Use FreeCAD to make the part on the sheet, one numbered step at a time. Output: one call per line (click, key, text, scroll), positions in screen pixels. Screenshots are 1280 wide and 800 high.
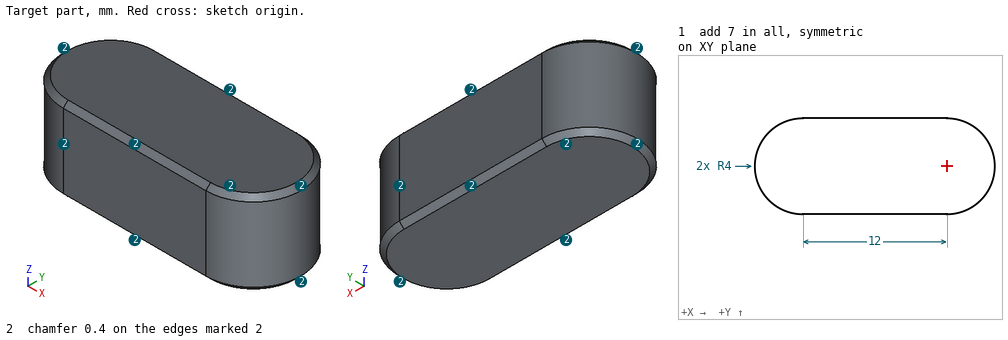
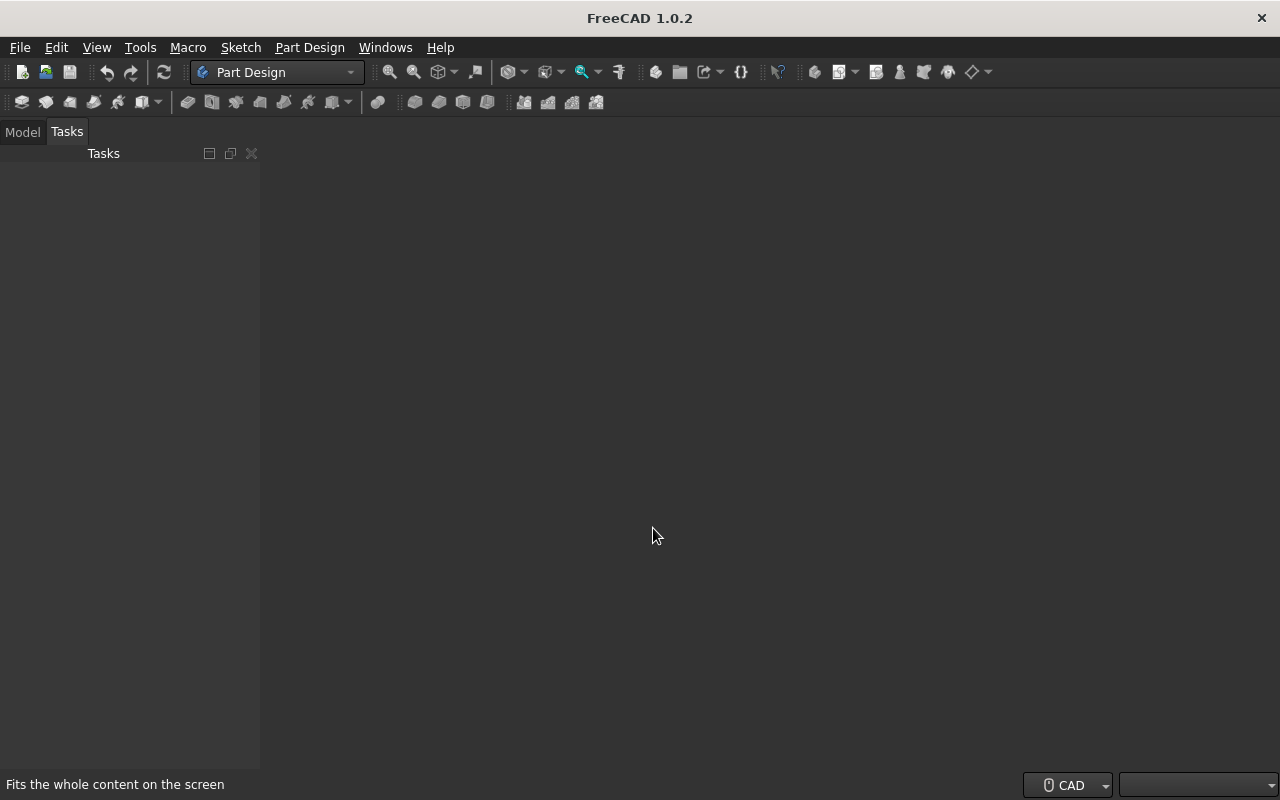
click(22, 72)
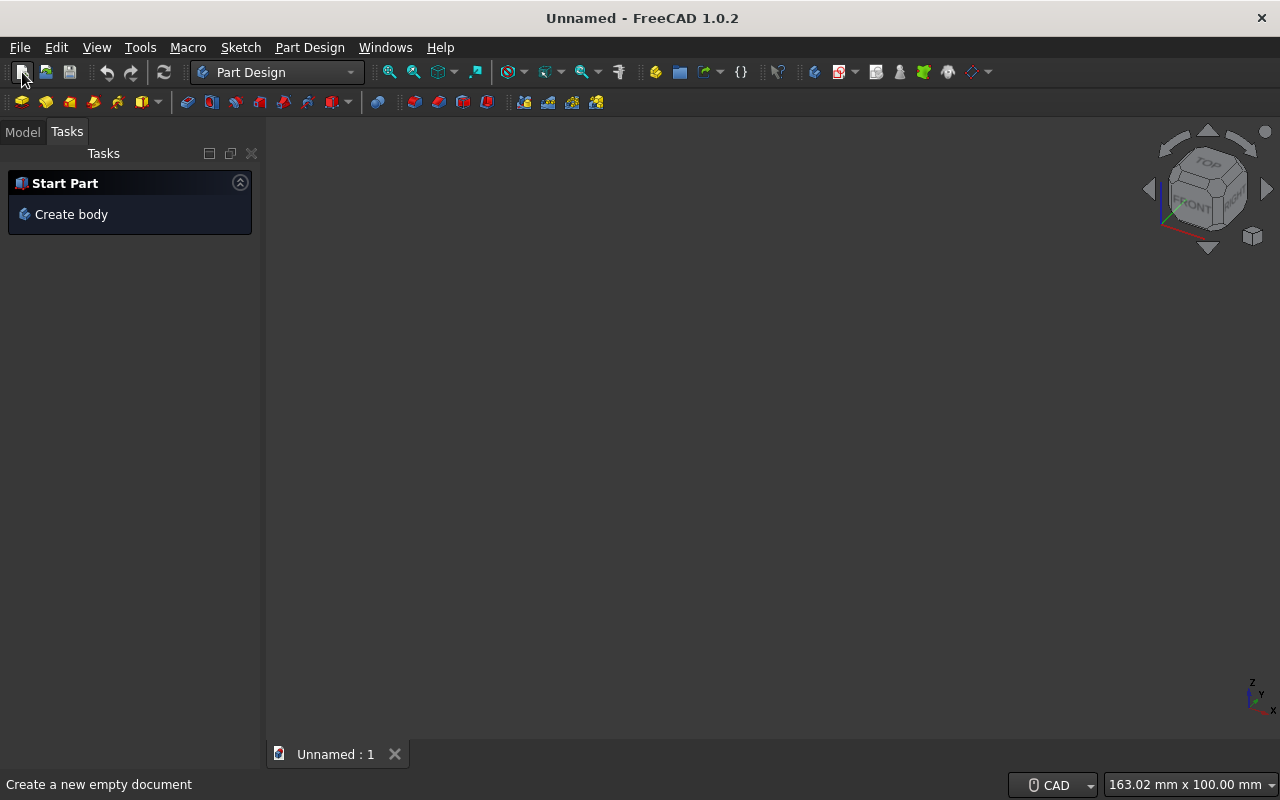
click(840, 72)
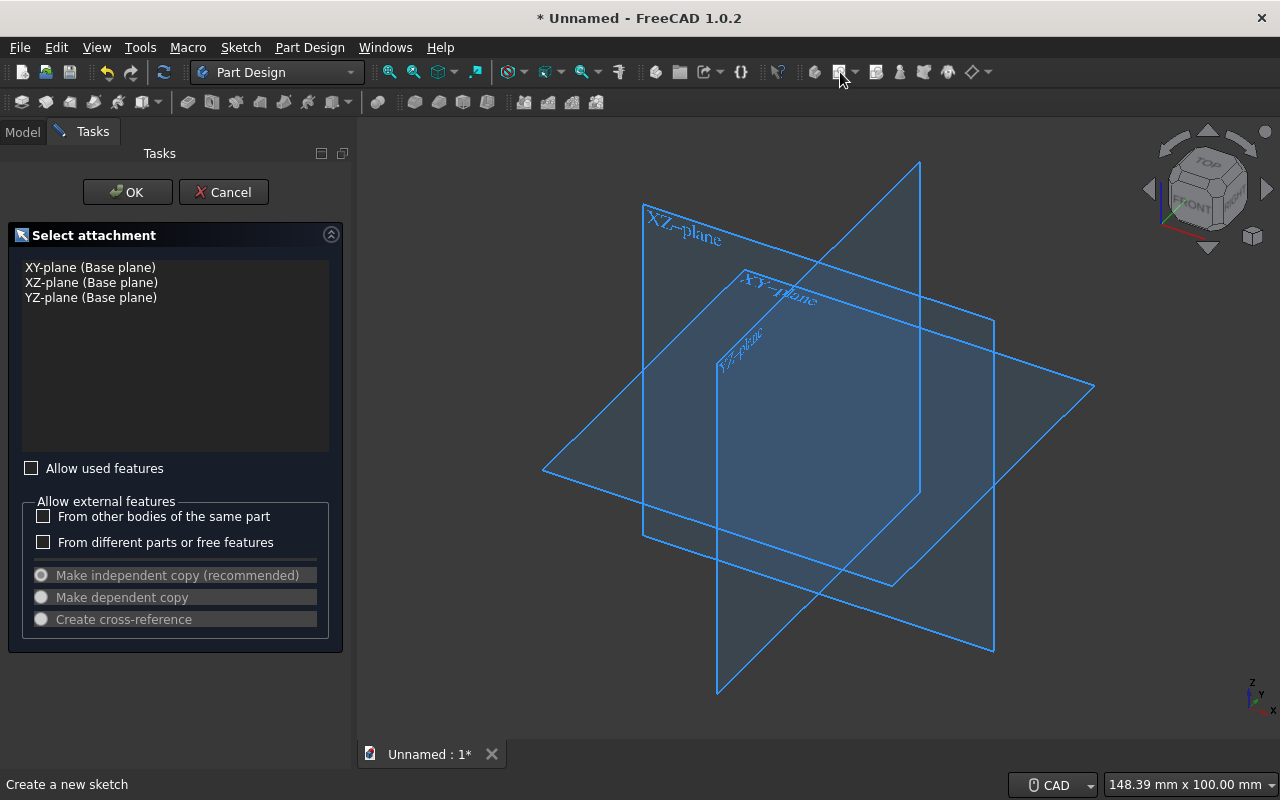
click(82, 268)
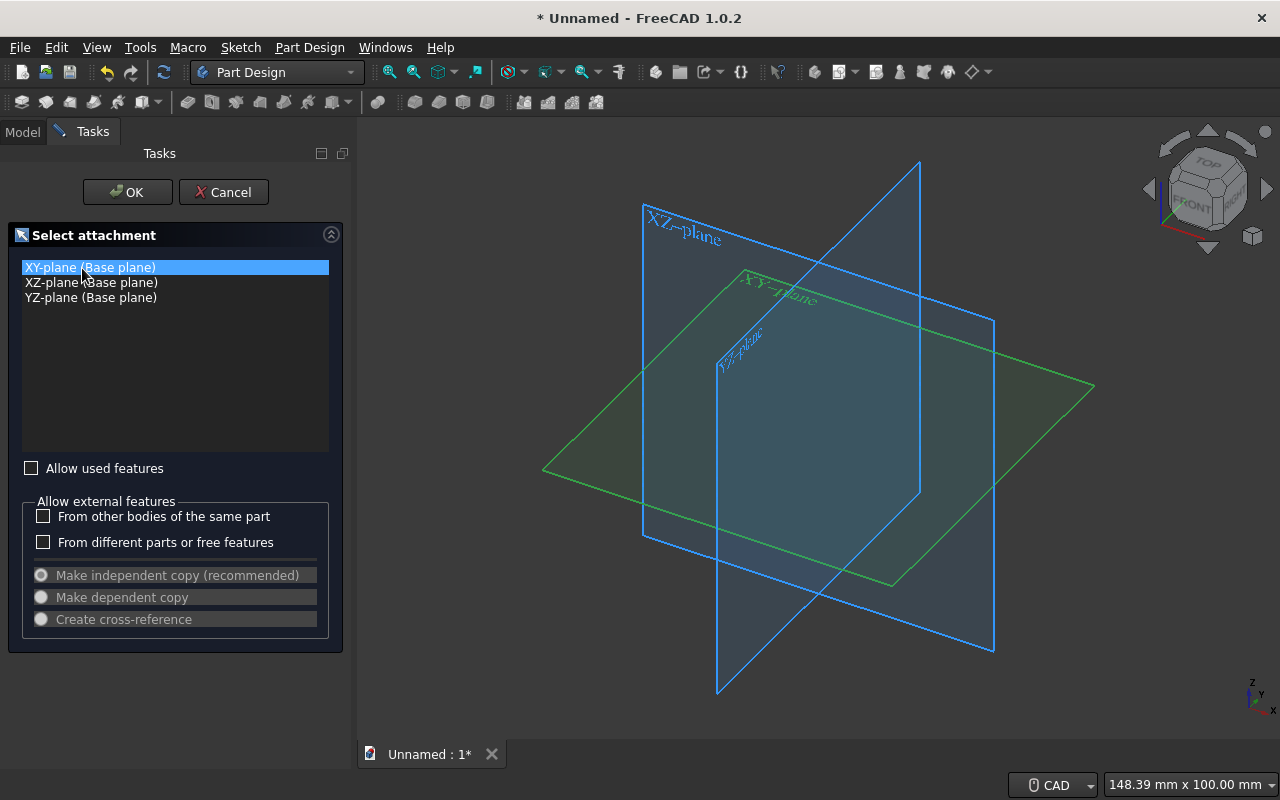
click(128, 192)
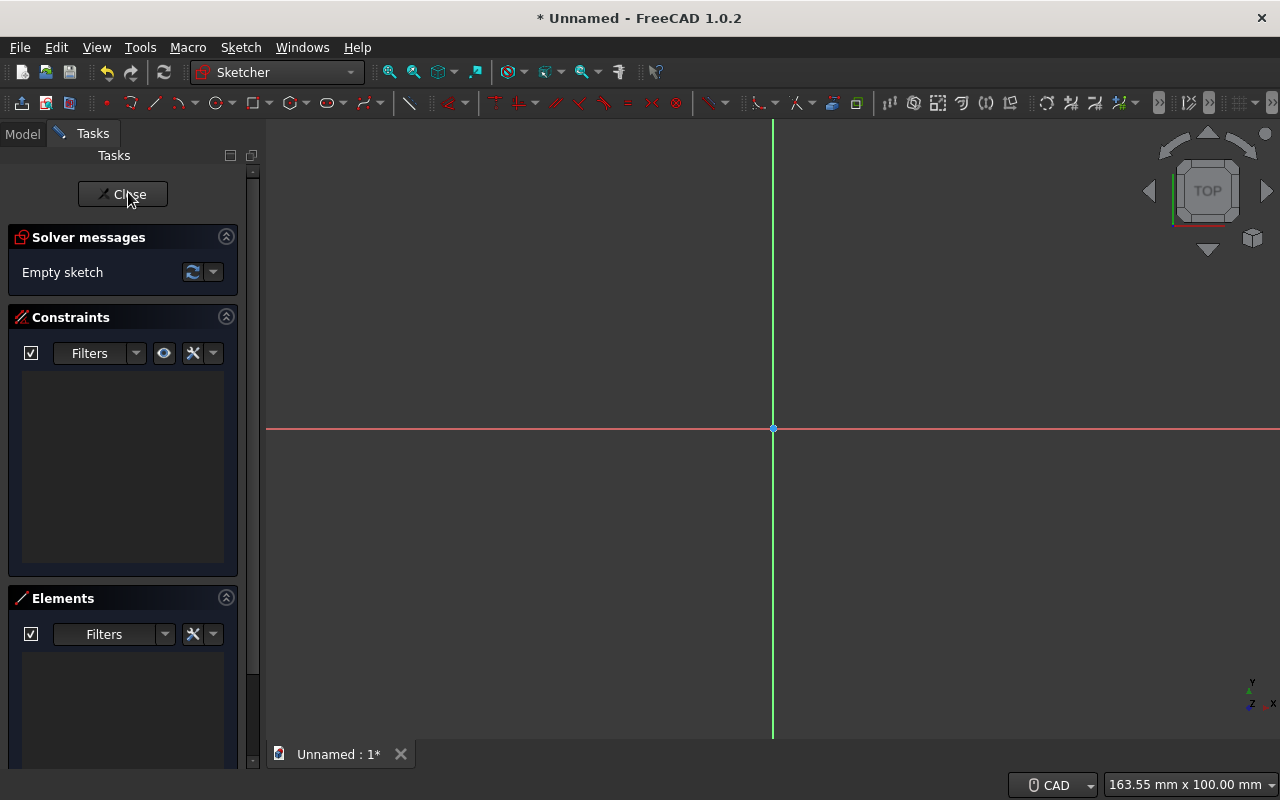
scroll(744, 429, up, 8)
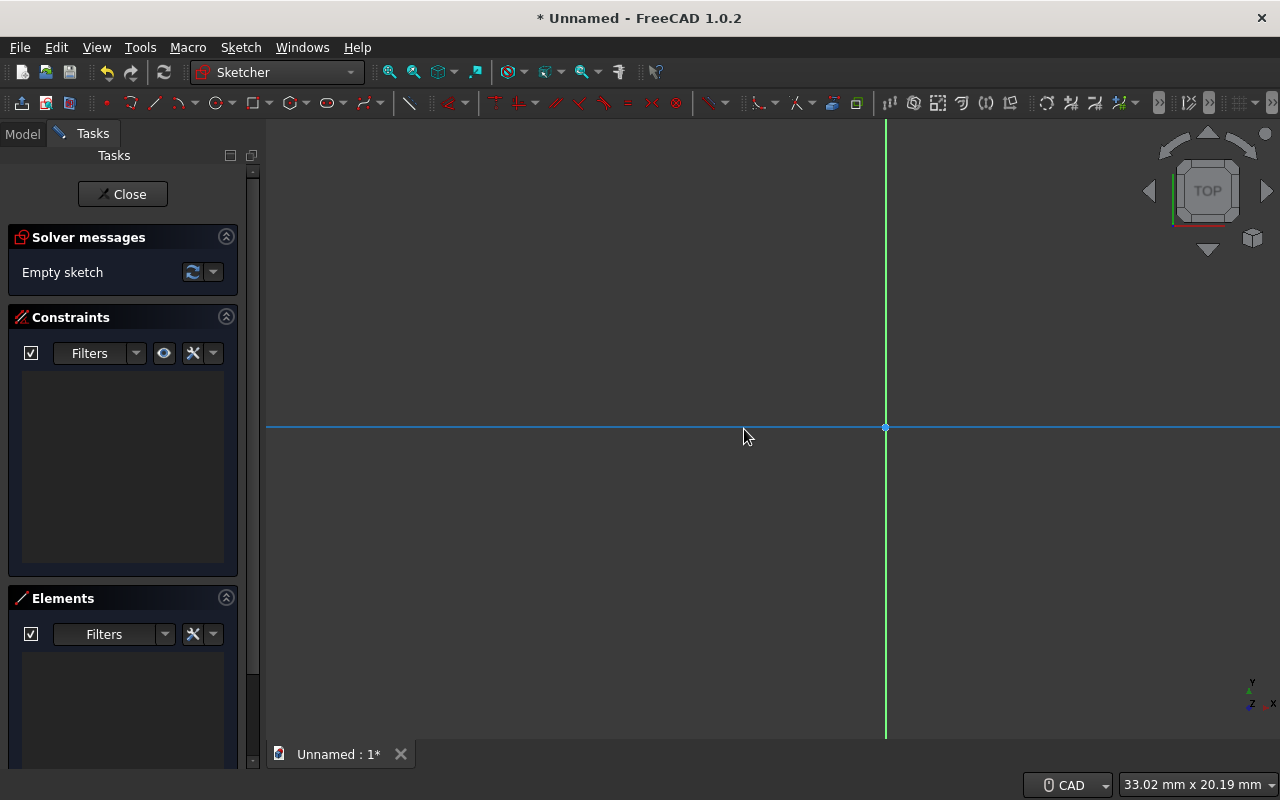
click(328, 104)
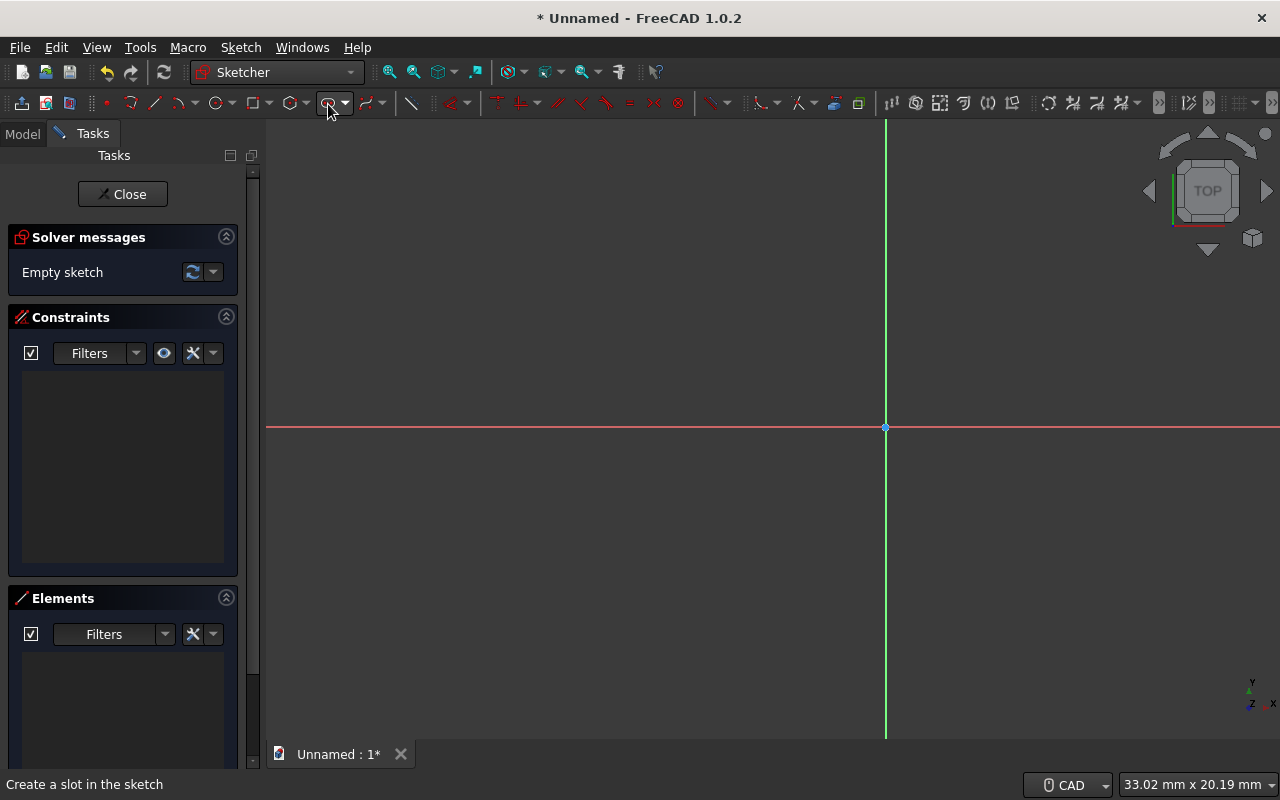
click(886, 427)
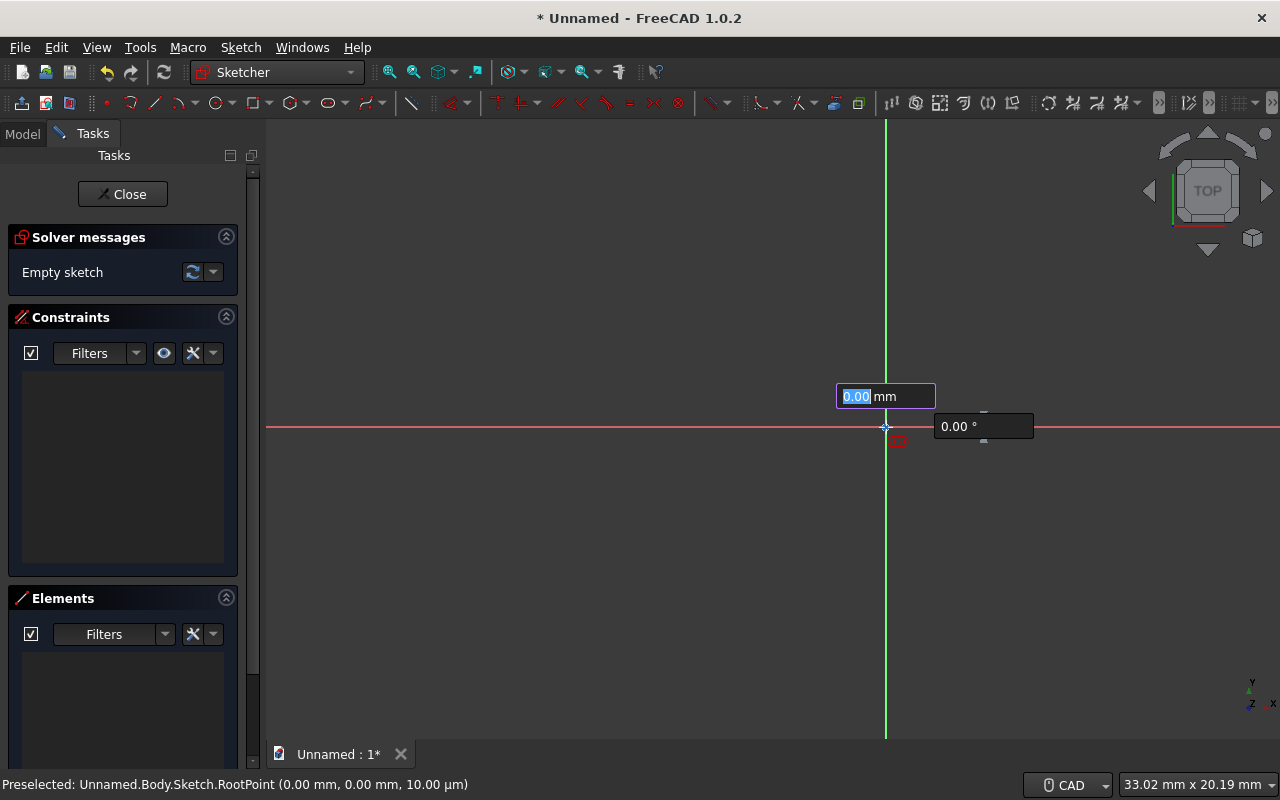
click(517, 418)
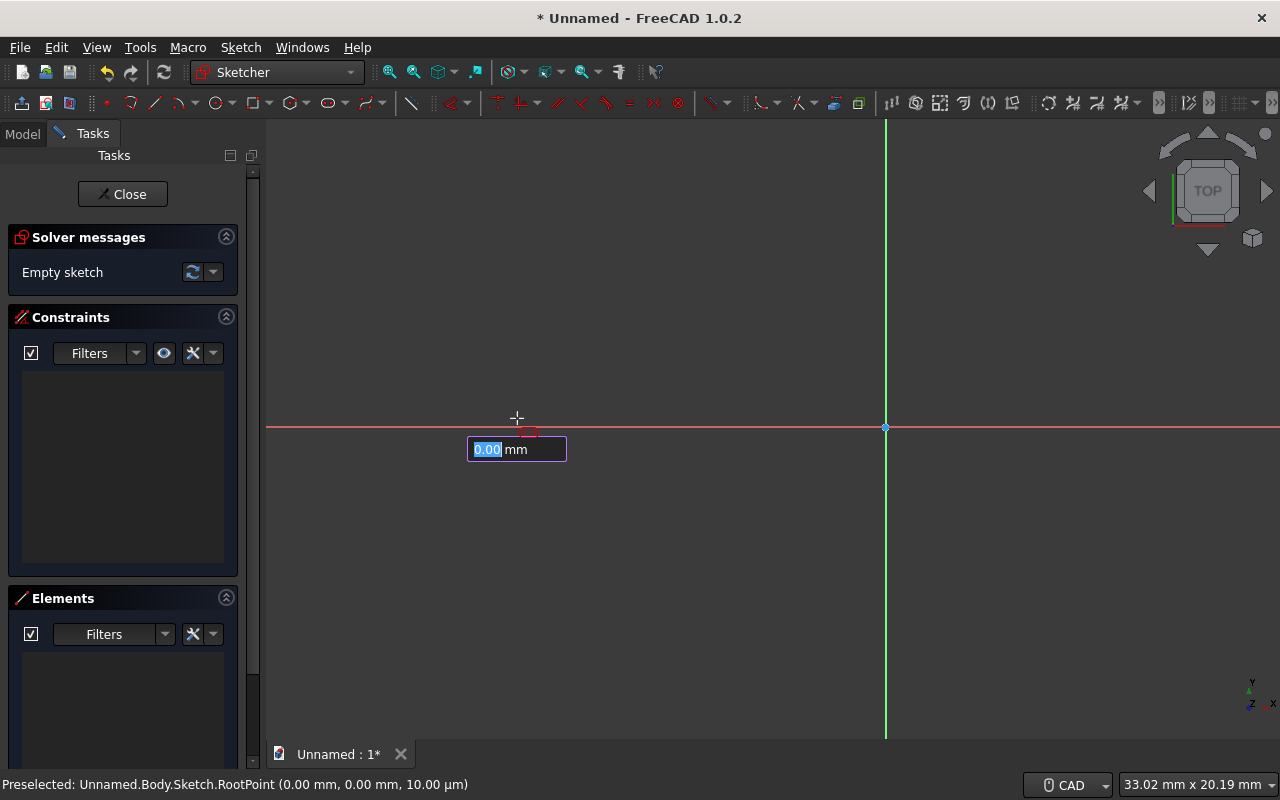
click(702, 304)
key(Escape)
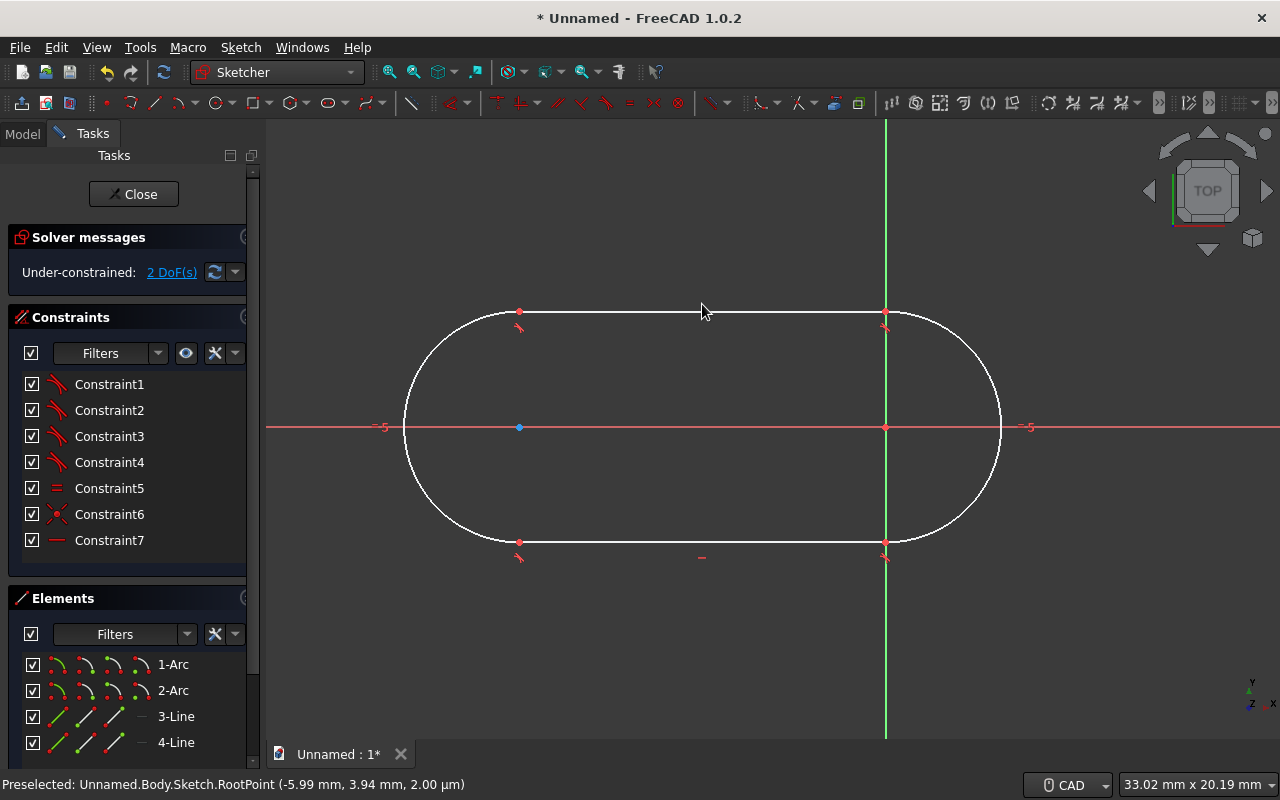
click(450, 104)